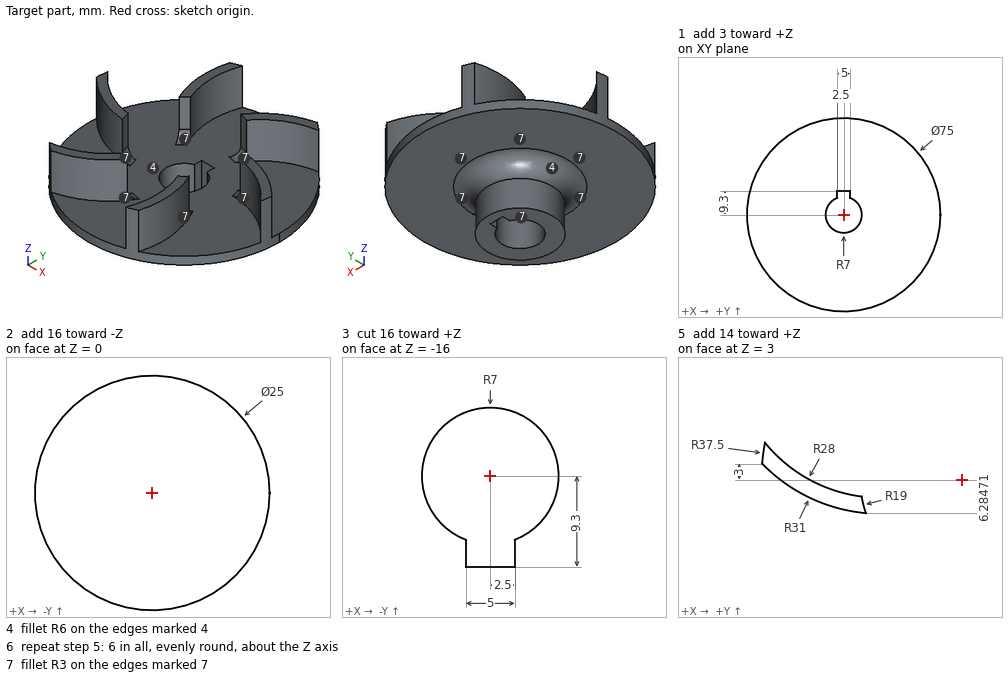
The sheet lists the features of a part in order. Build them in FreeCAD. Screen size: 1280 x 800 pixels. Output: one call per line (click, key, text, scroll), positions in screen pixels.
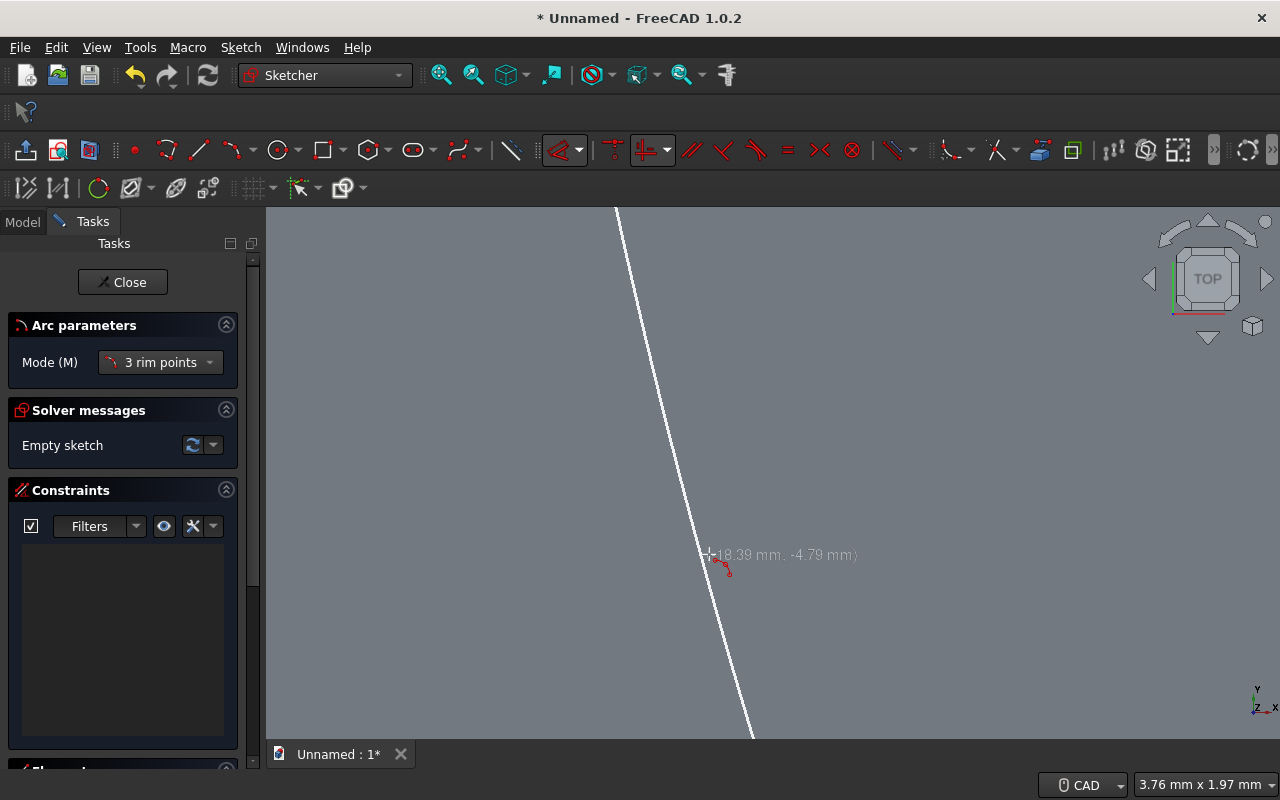
click(701, 550)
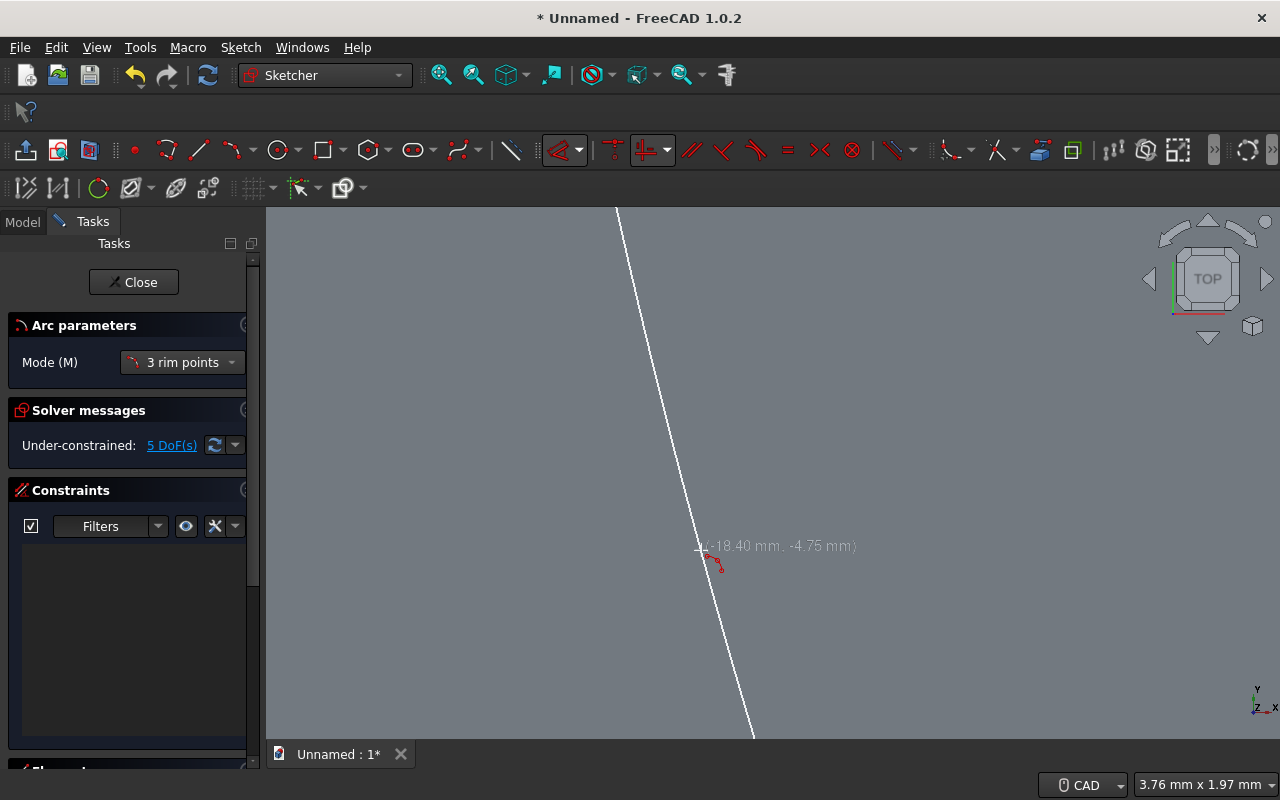
scroll(710, 557, down, 14)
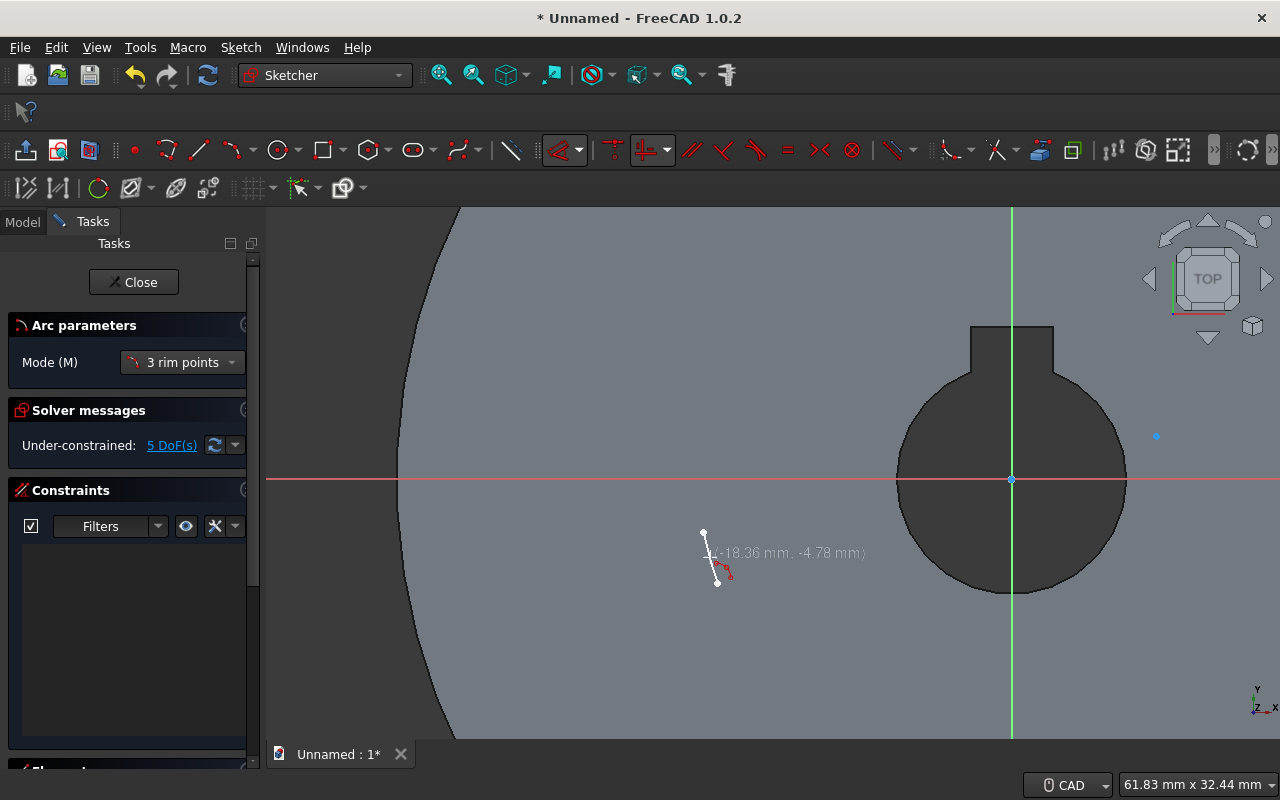
click(704, 533)
click(407, 366)
click(510, 459)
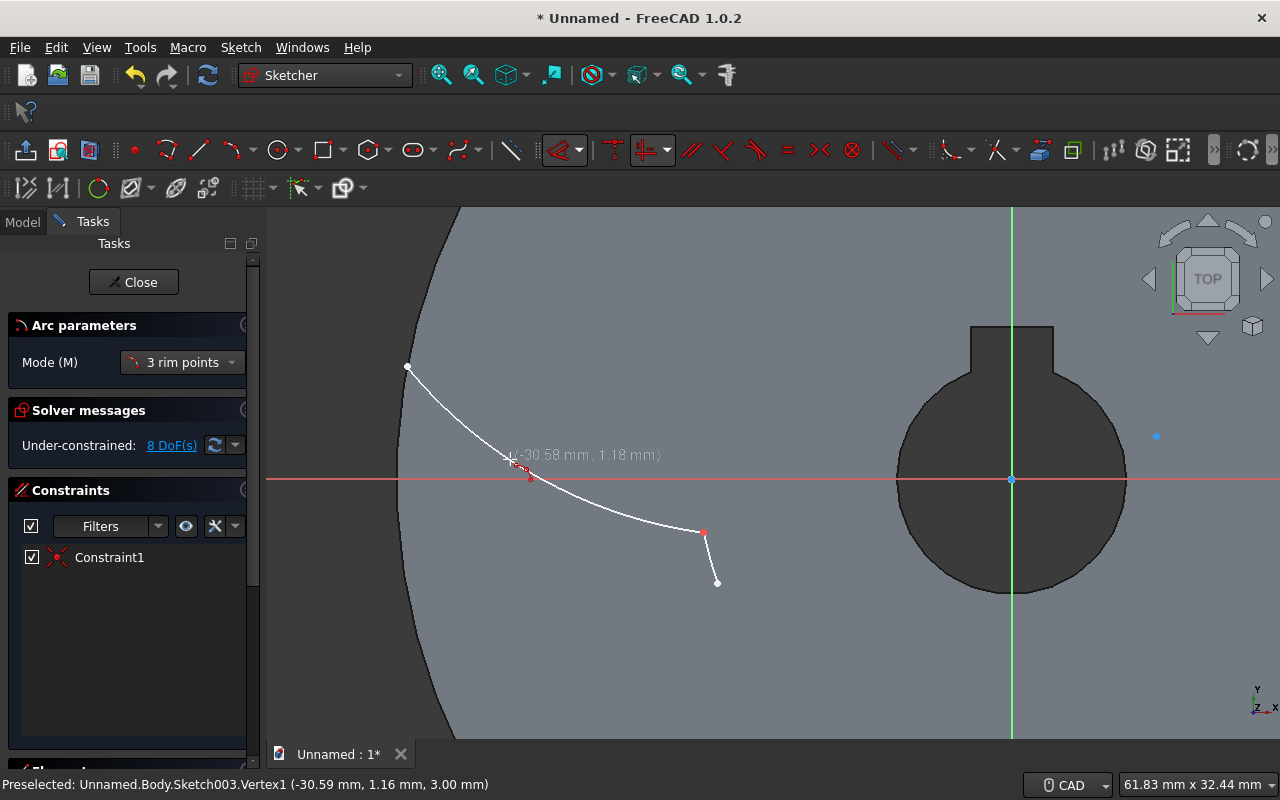
click(407, 367)
click(399, 430)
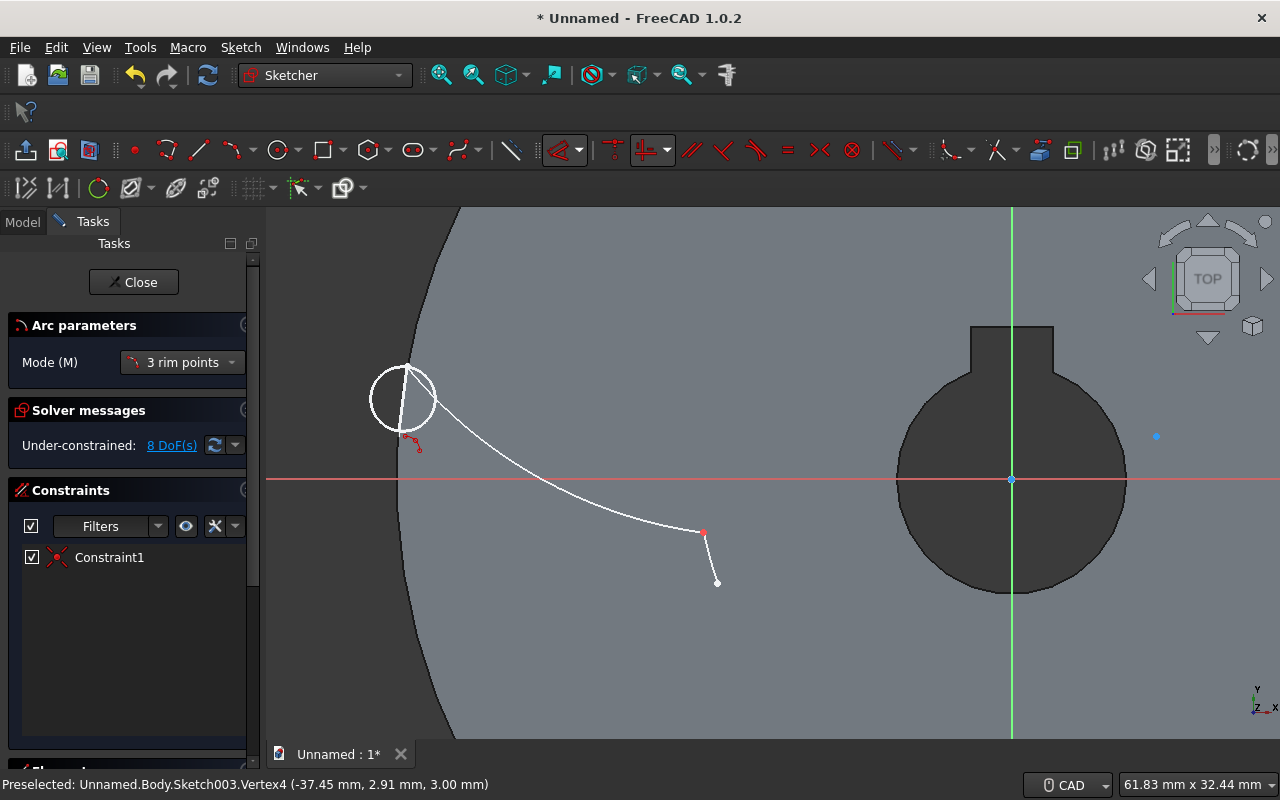
scroll(402, 398, up, 15)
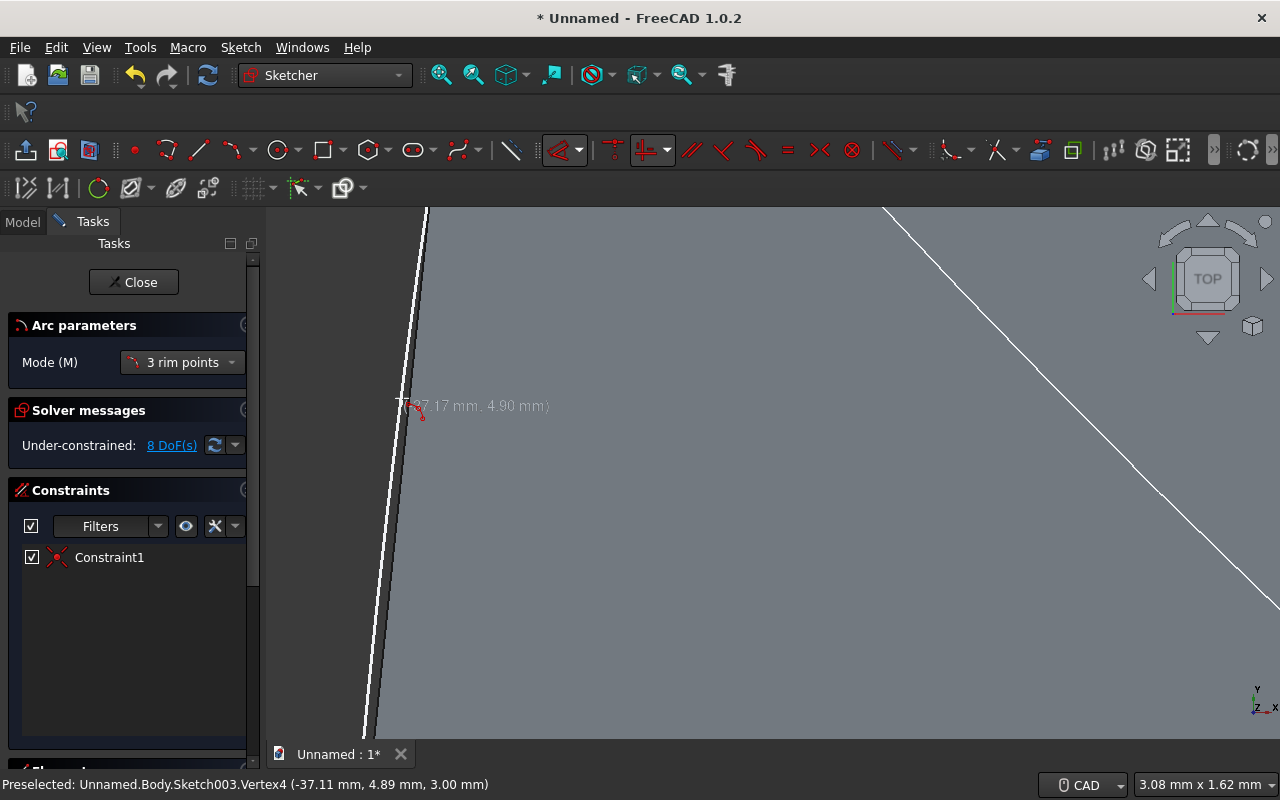
click(400, 388)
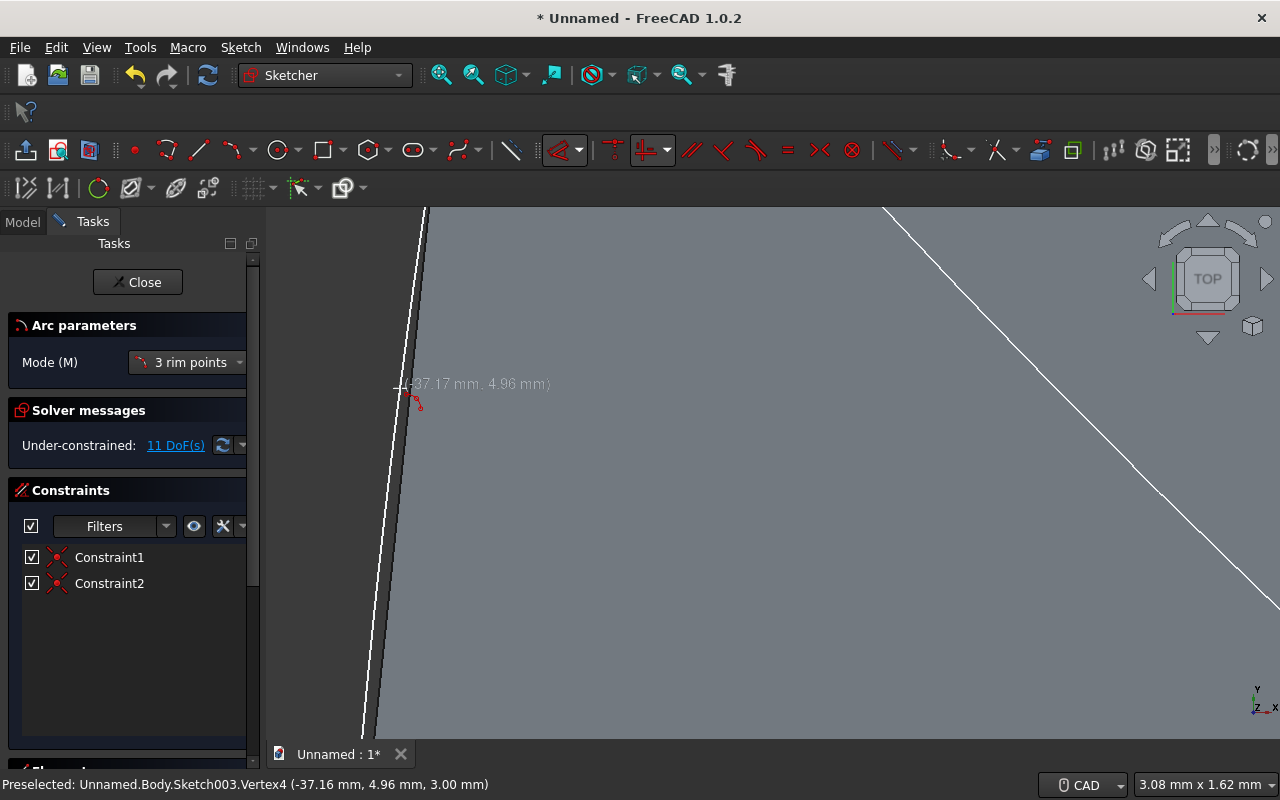
scroll(402, 397, down, 15)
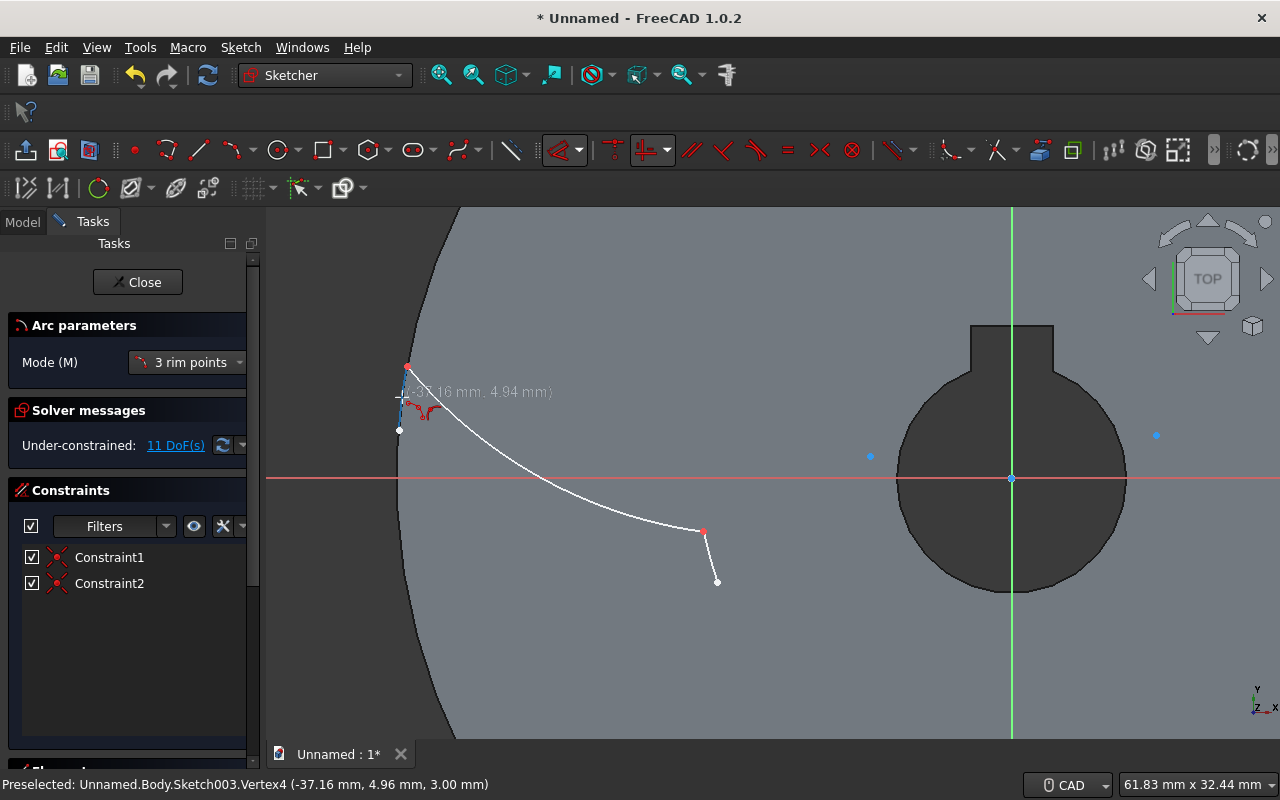
click(399, 430)
click(718, 583)
click(544, 534)
key(Escape)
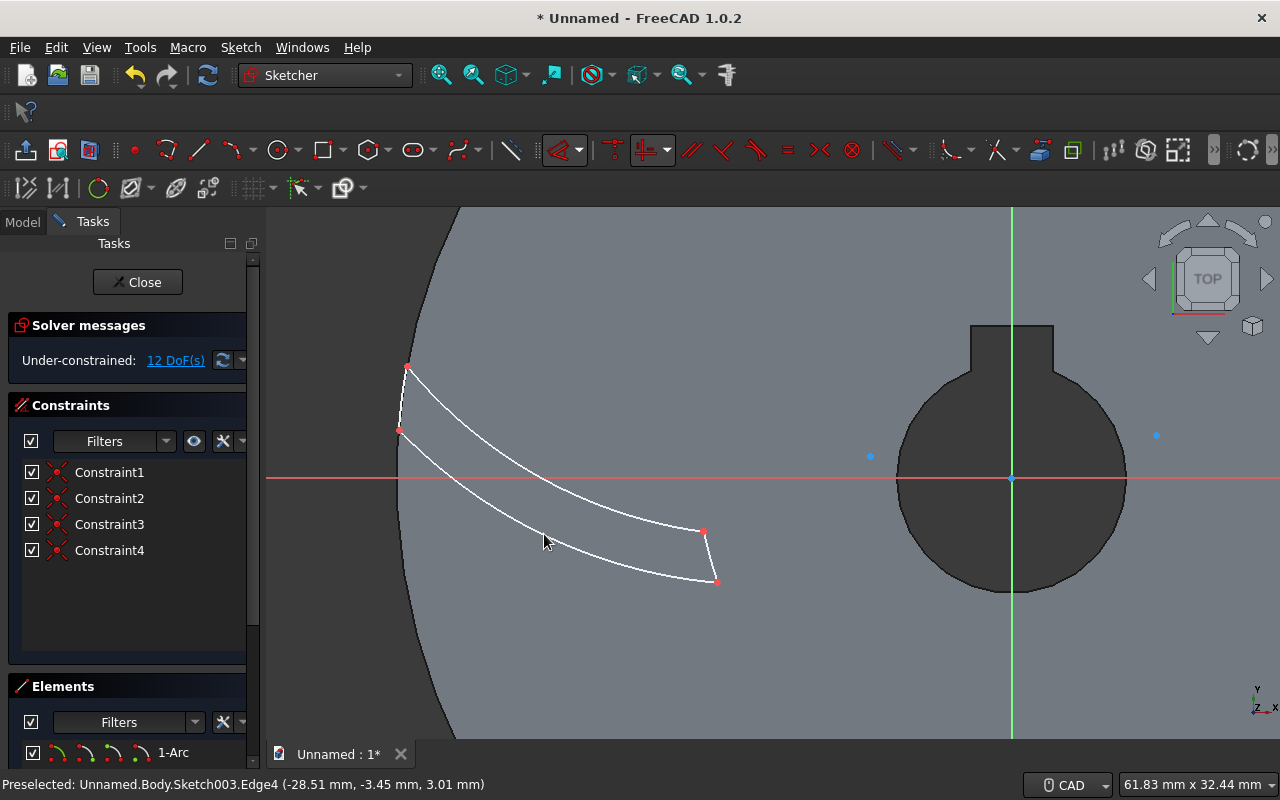
click(708, 547)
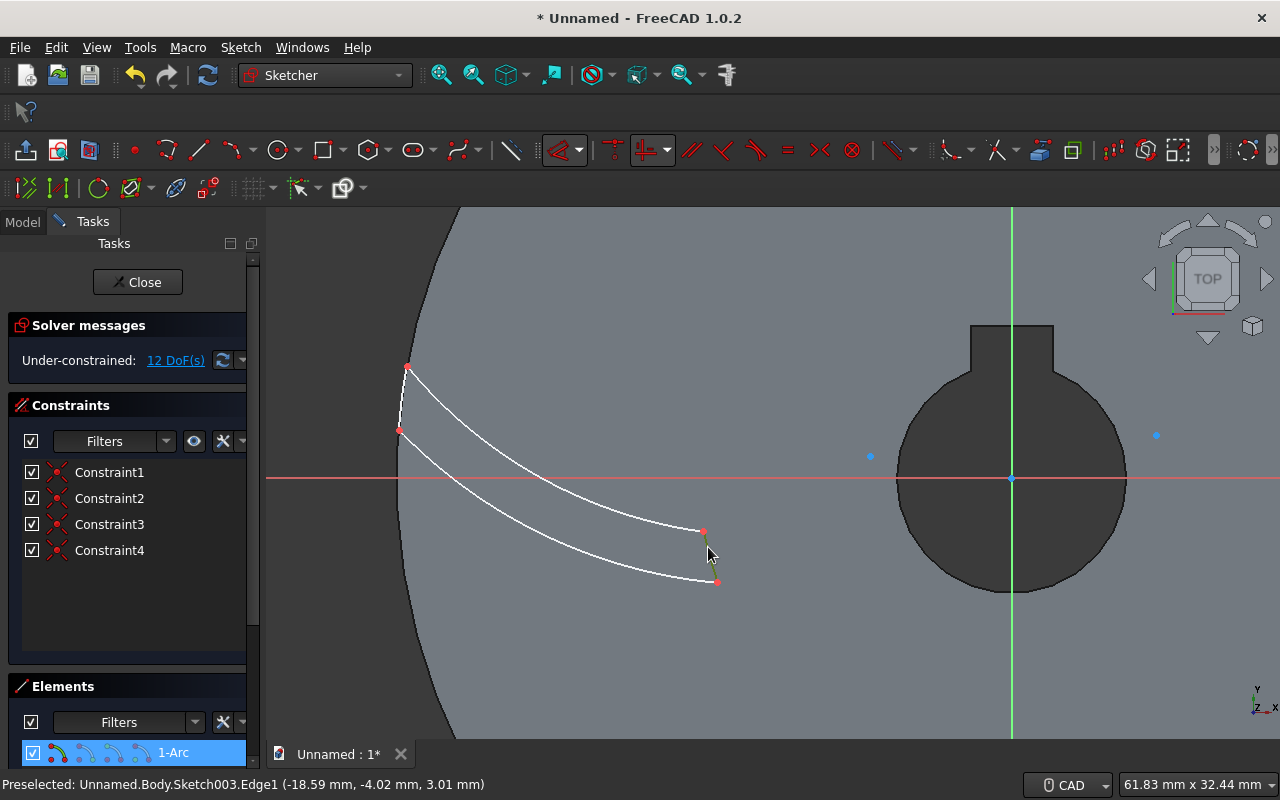
click(404, 385)